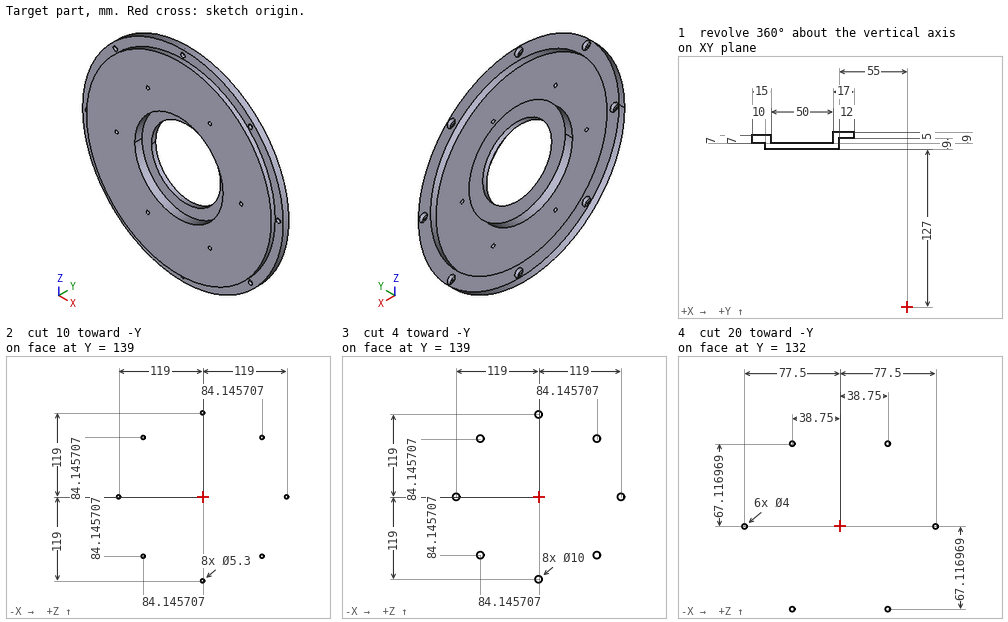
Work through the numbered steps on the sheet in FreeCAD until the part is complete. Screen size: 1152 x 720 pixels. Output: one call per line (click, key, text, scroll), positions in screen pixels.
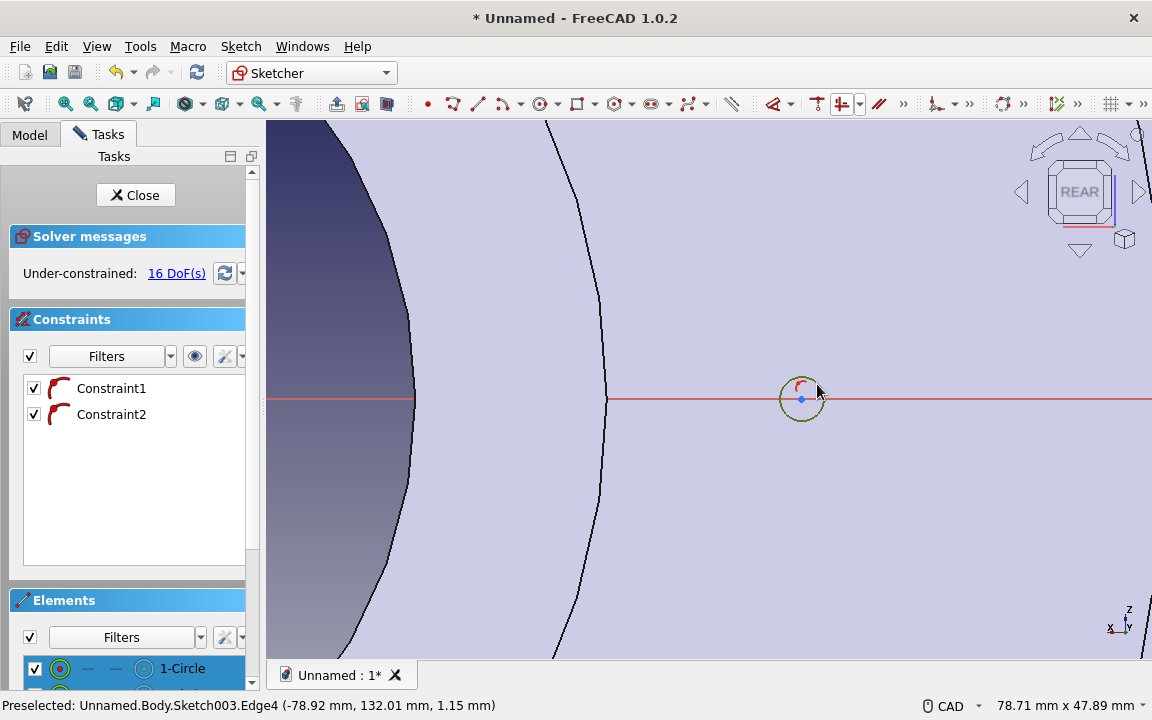
scroll(820, 387, down, 8)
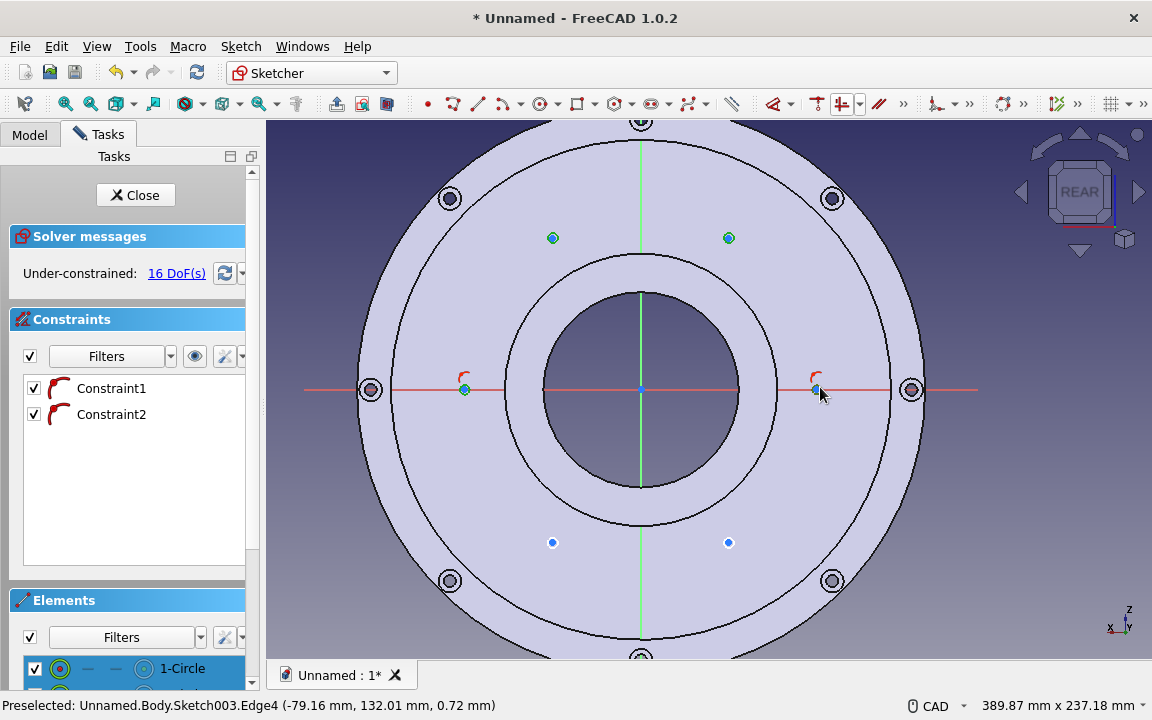
scroll(732, 539, up, 6)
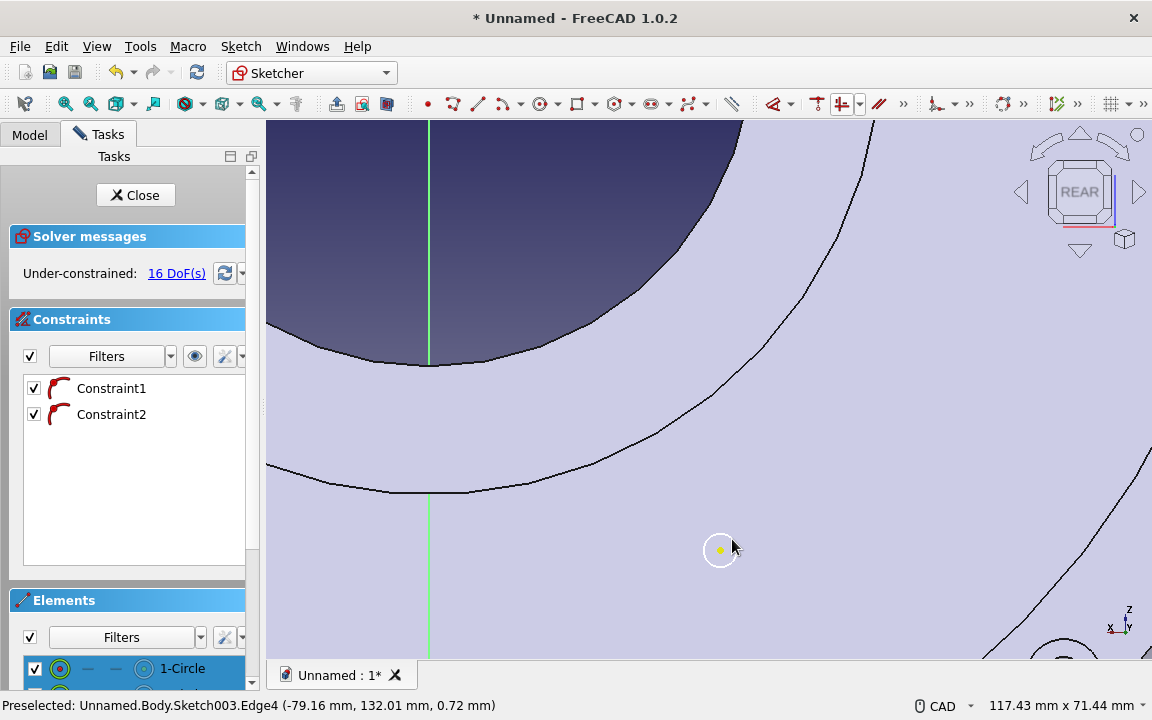
click(732, 539)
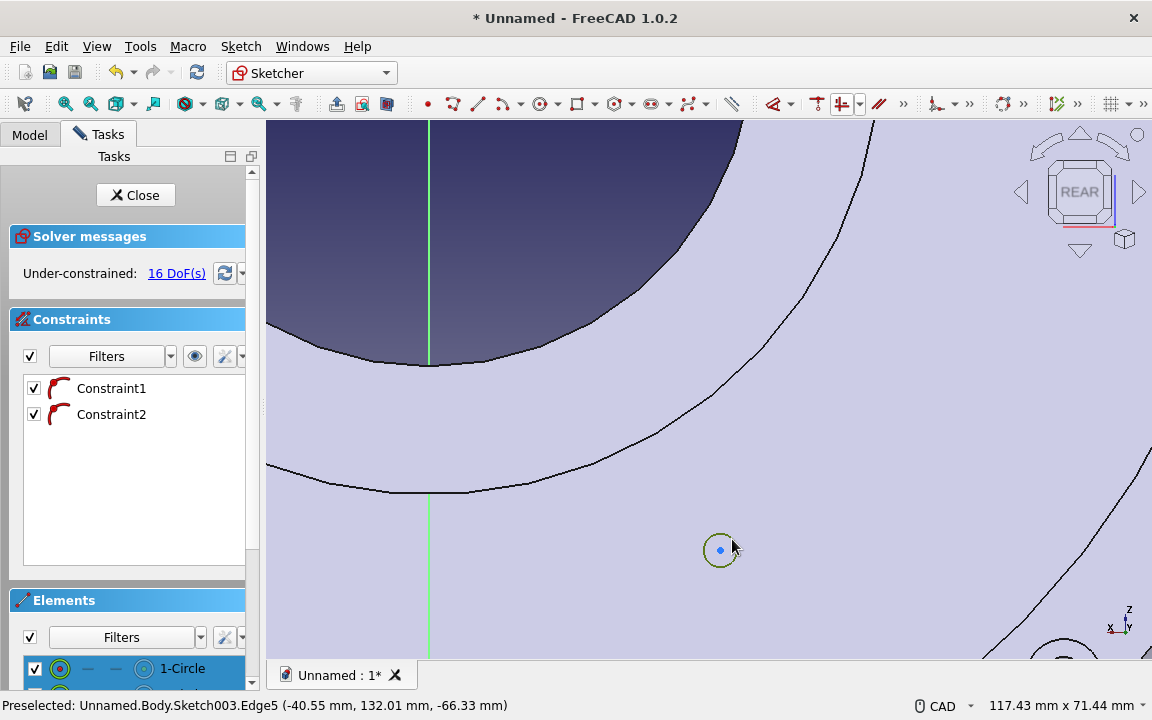
scroll(732, 539, down, 6)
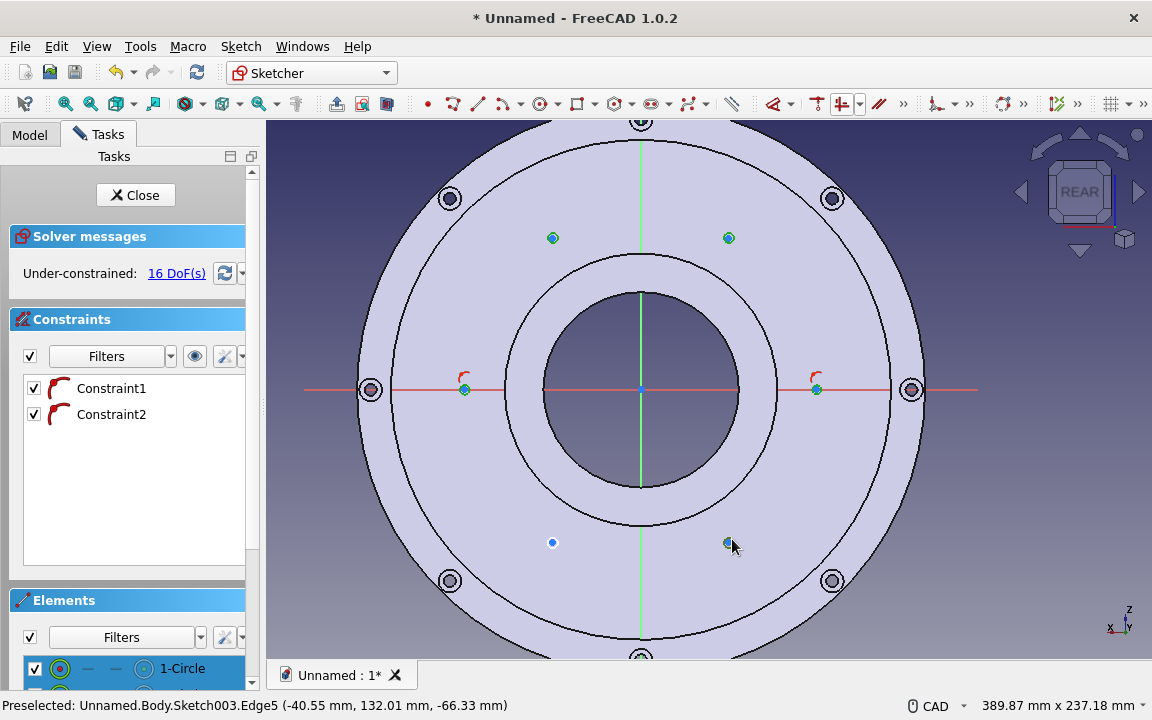
scroll(556, 539, up, 6)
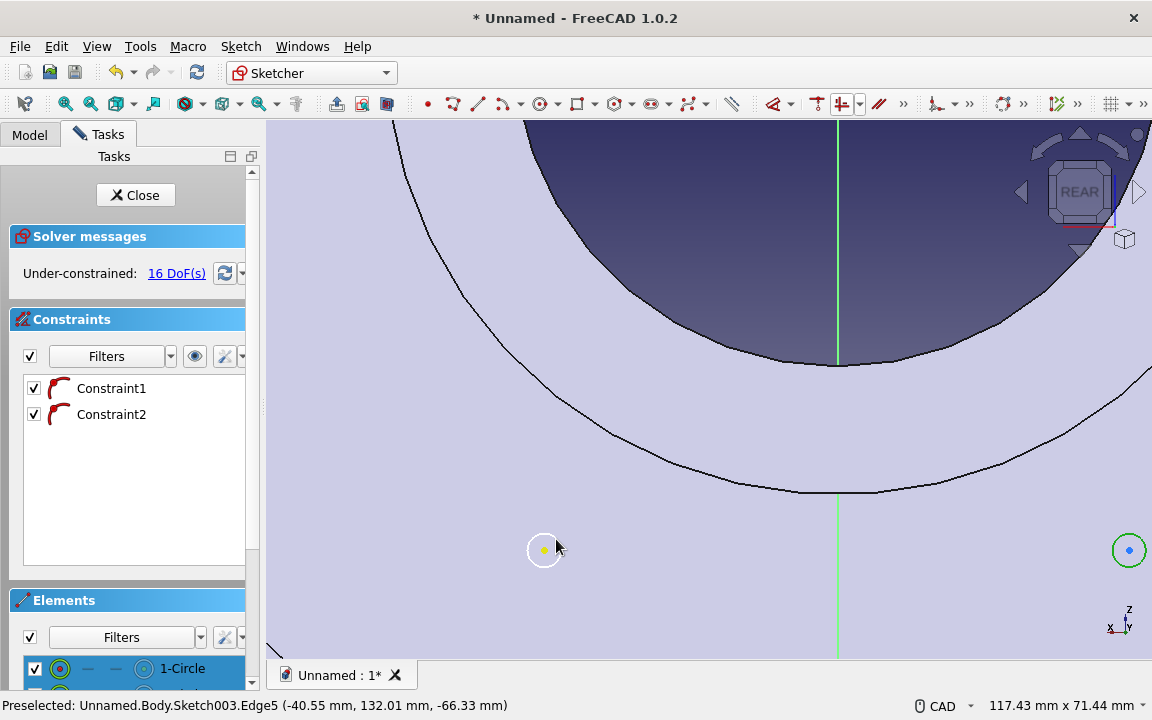
click(556, 539)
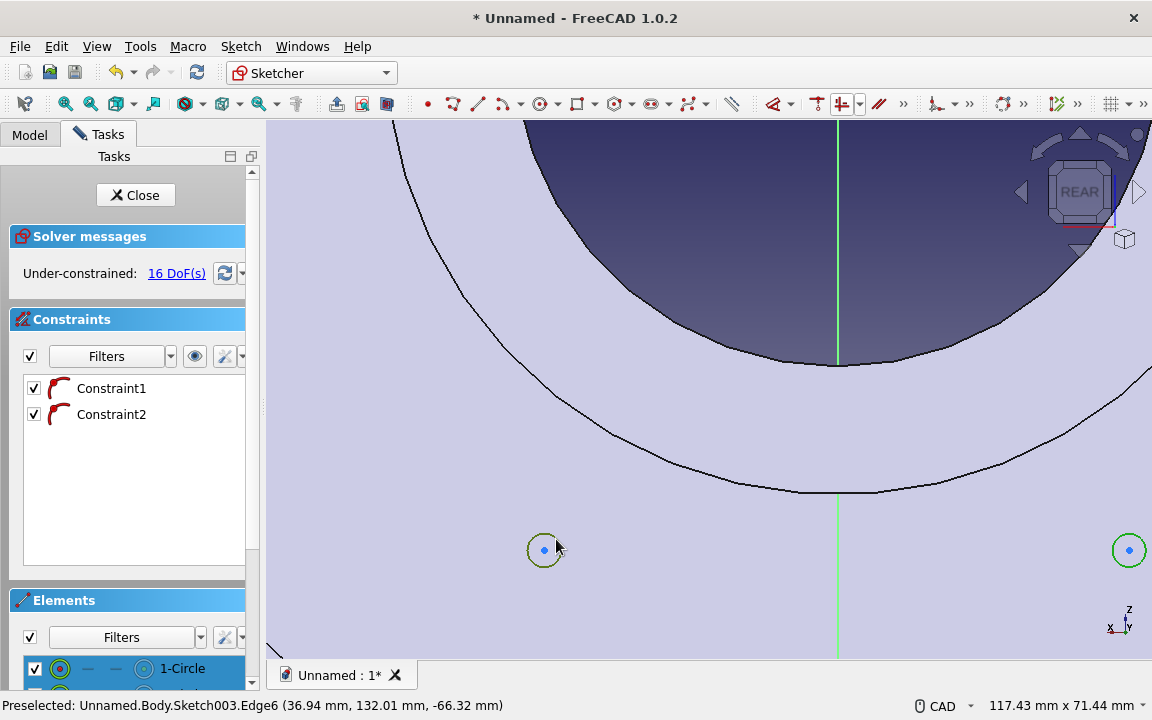
key(e)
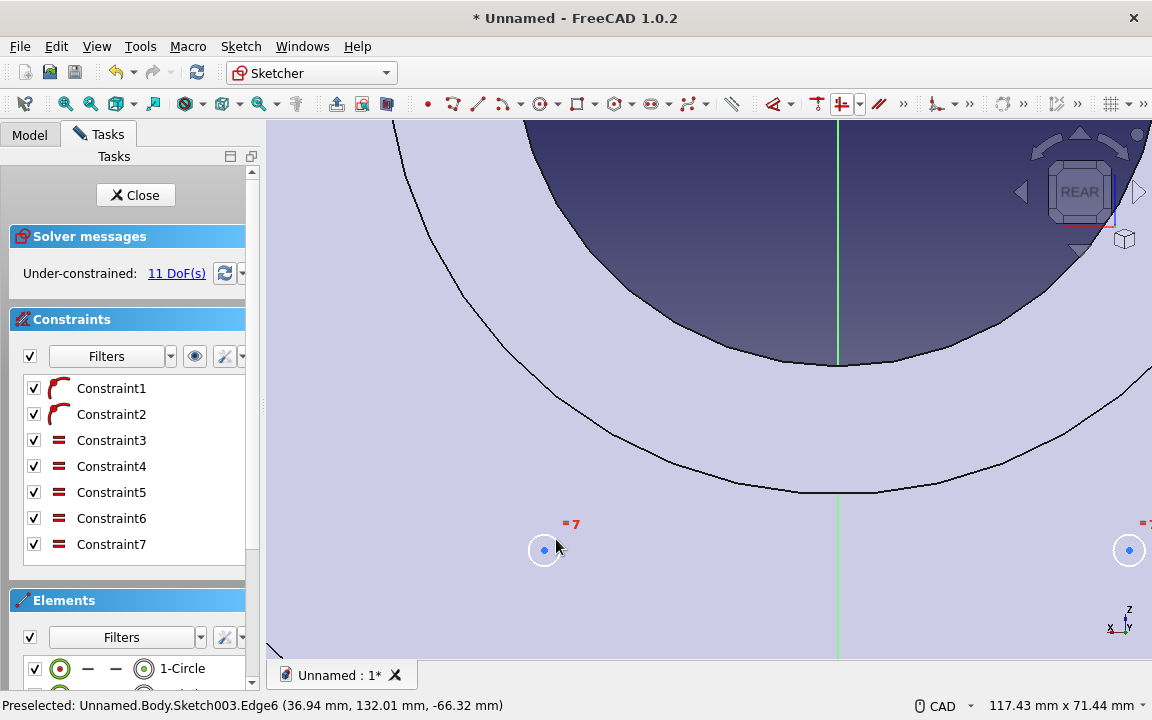
scroll(555, 539, down, 6)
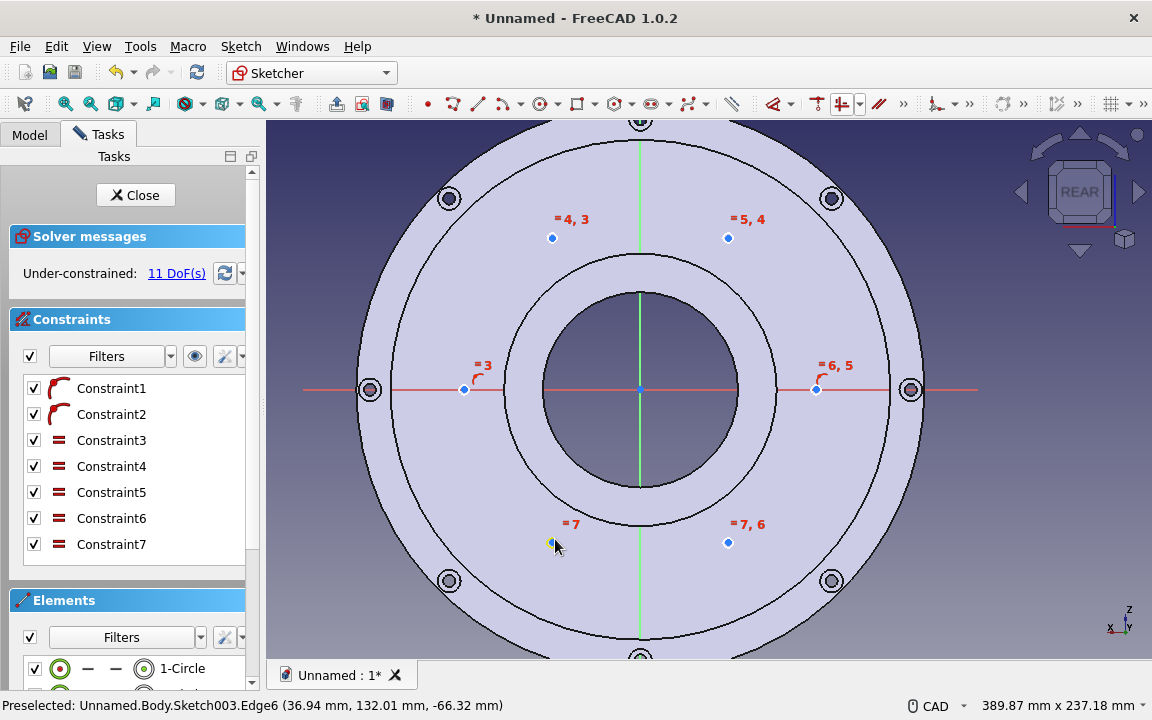
click(552, 238)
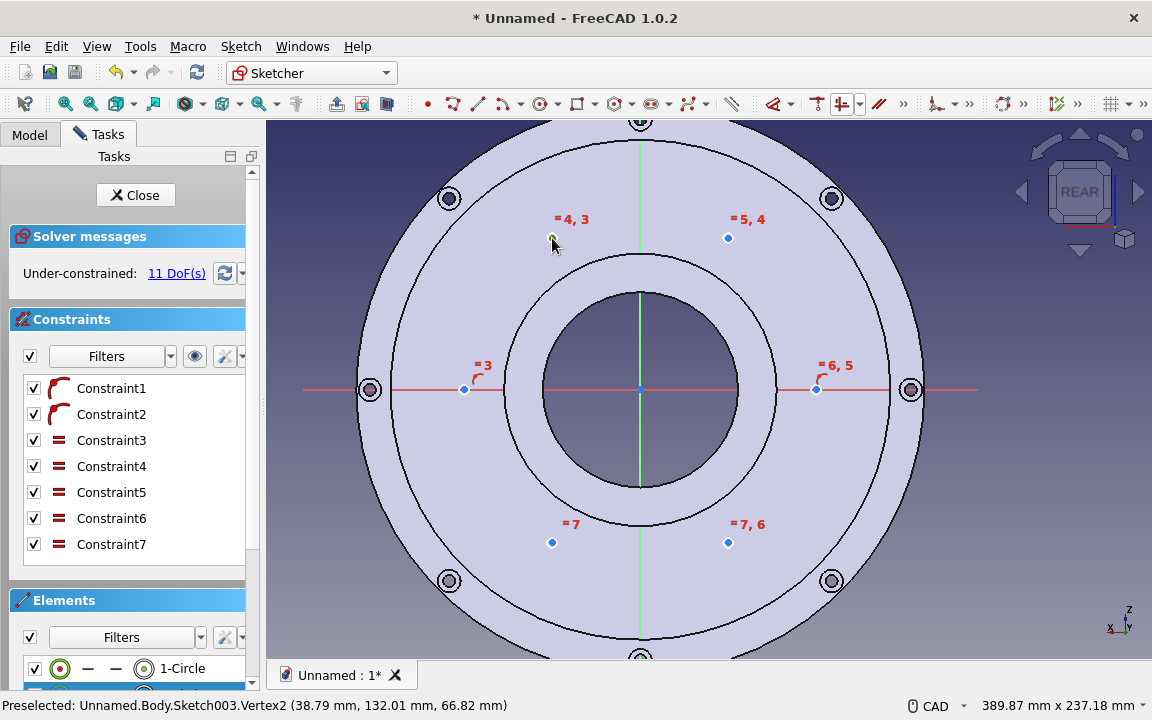
click(728, 238)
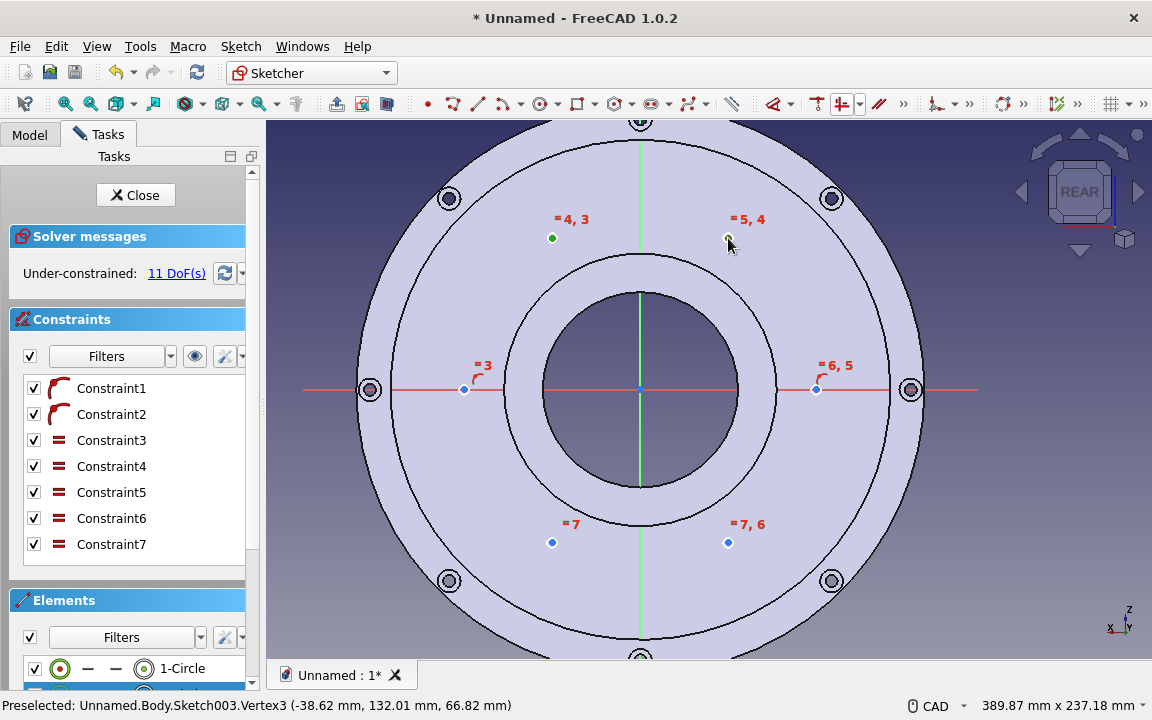
click(860, 104)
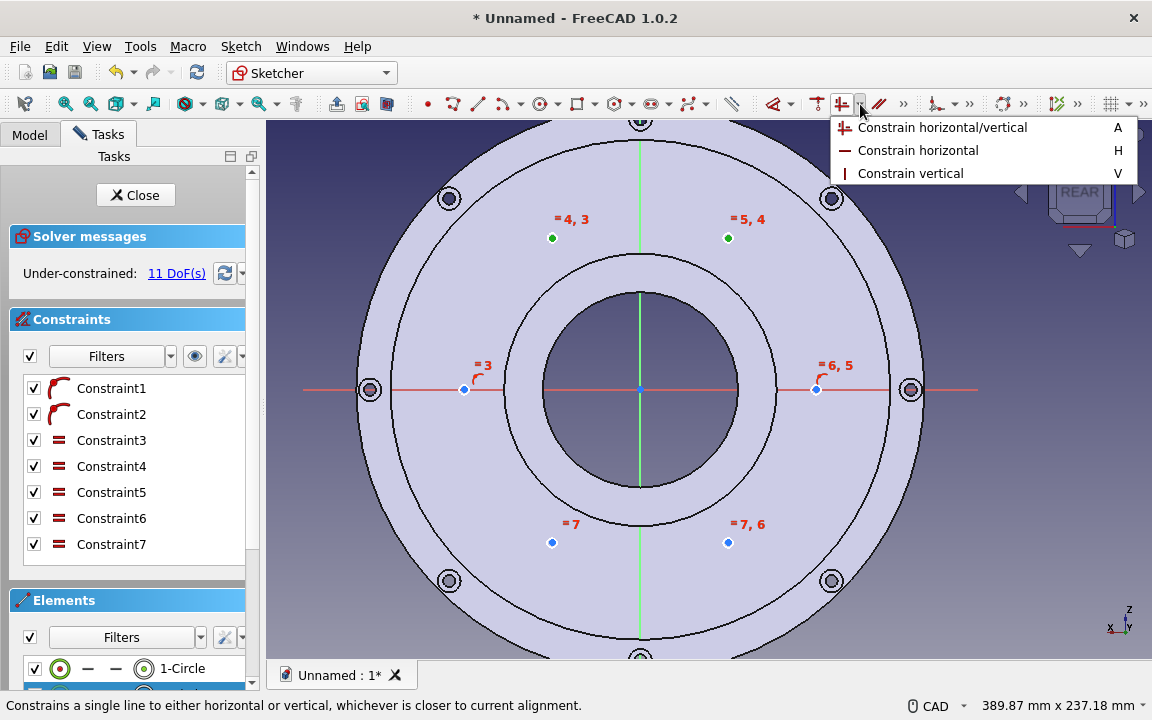
click(984, 150)